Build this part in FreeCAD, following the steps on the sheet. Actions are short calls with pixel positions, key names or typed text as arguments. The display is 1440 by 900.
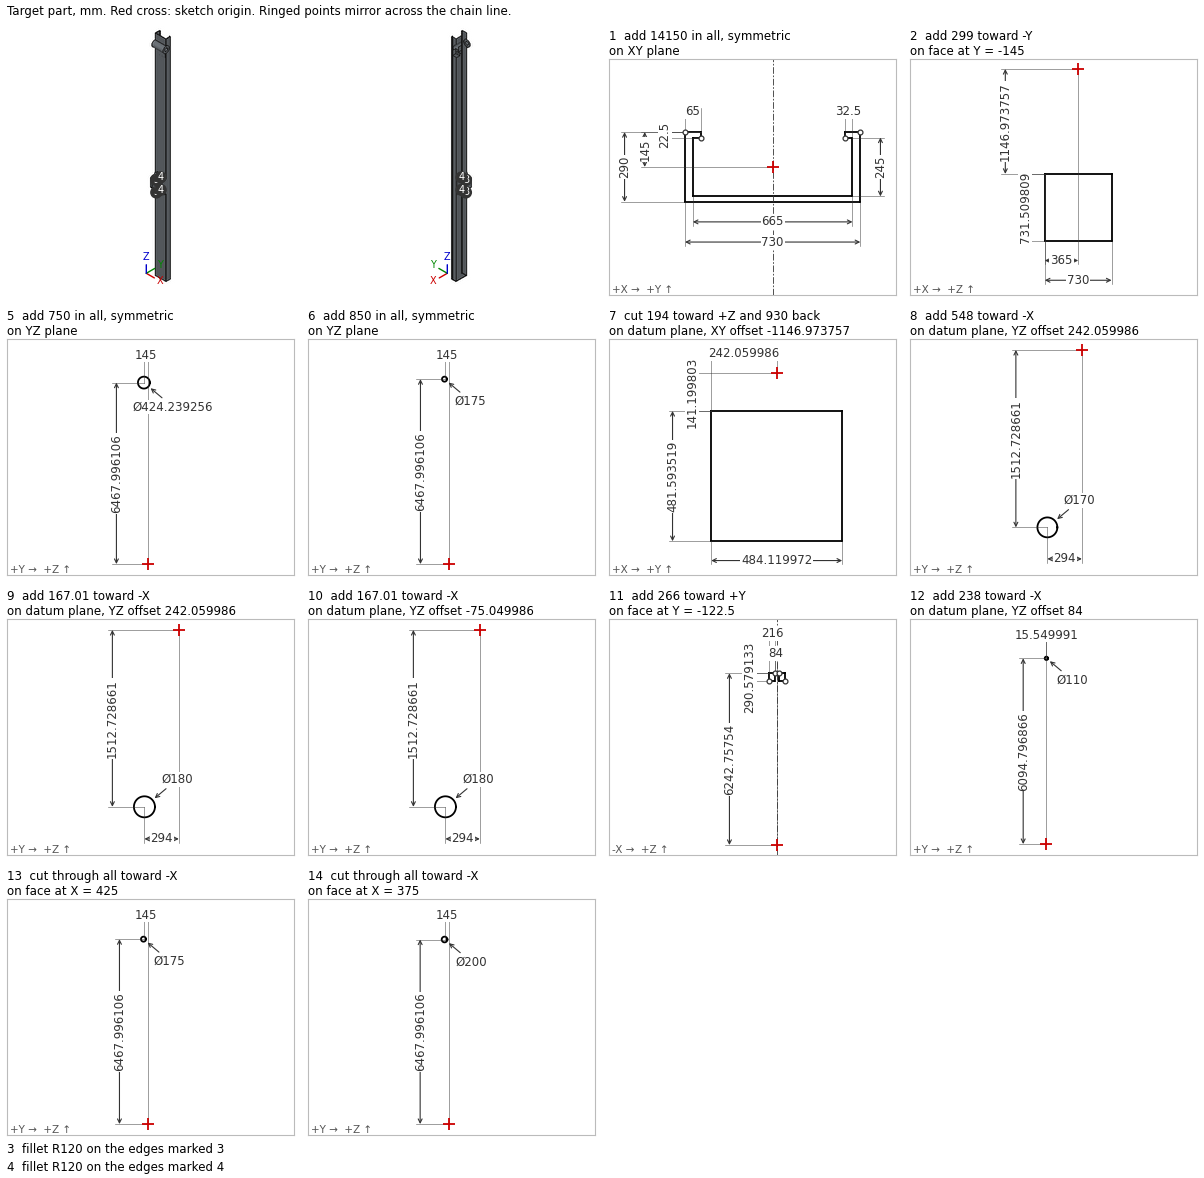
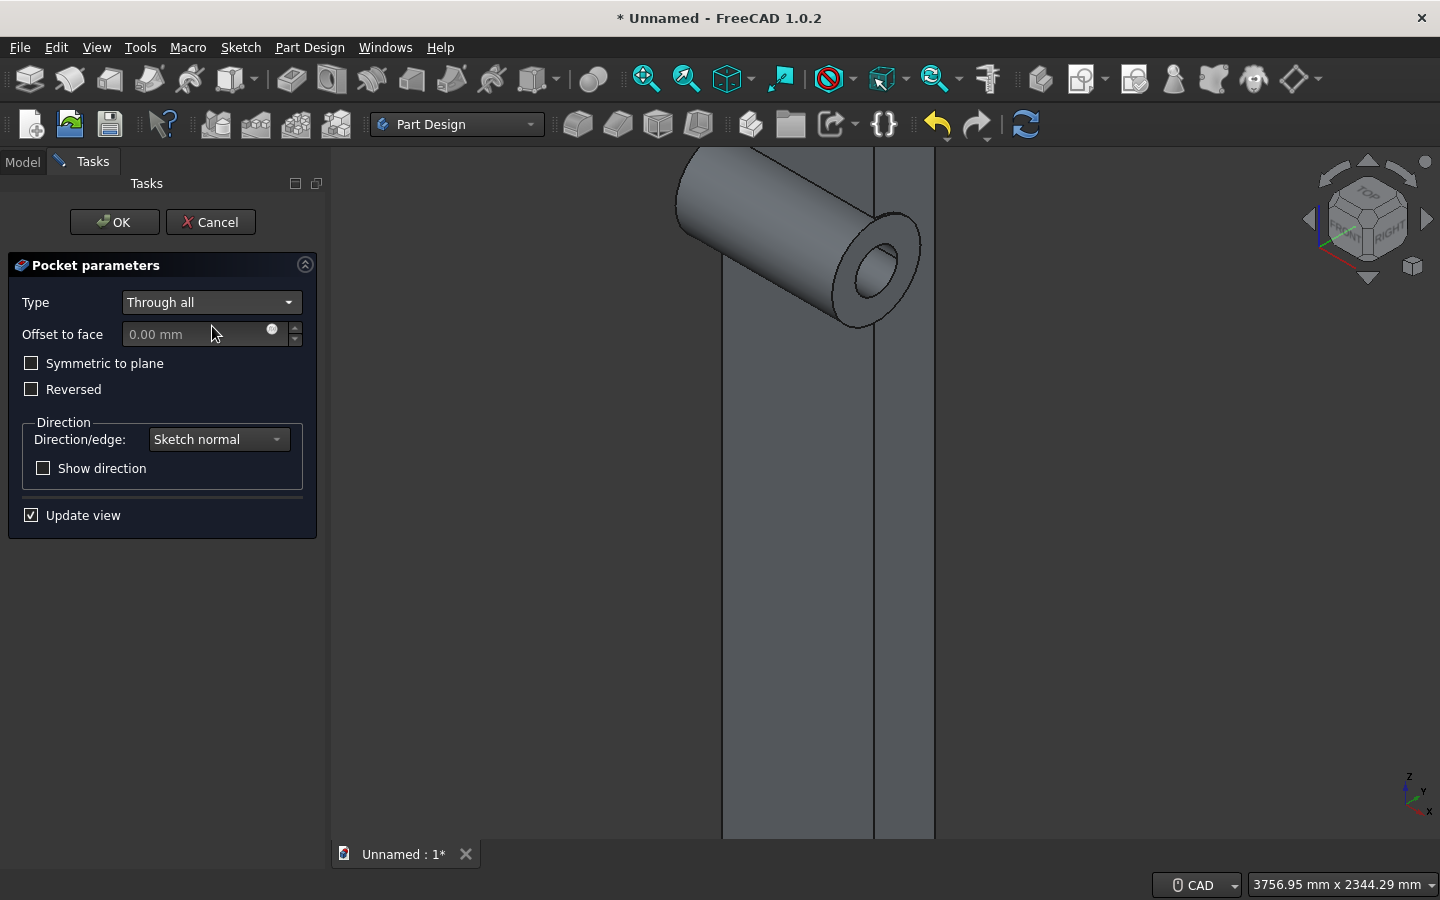
click(115, 222)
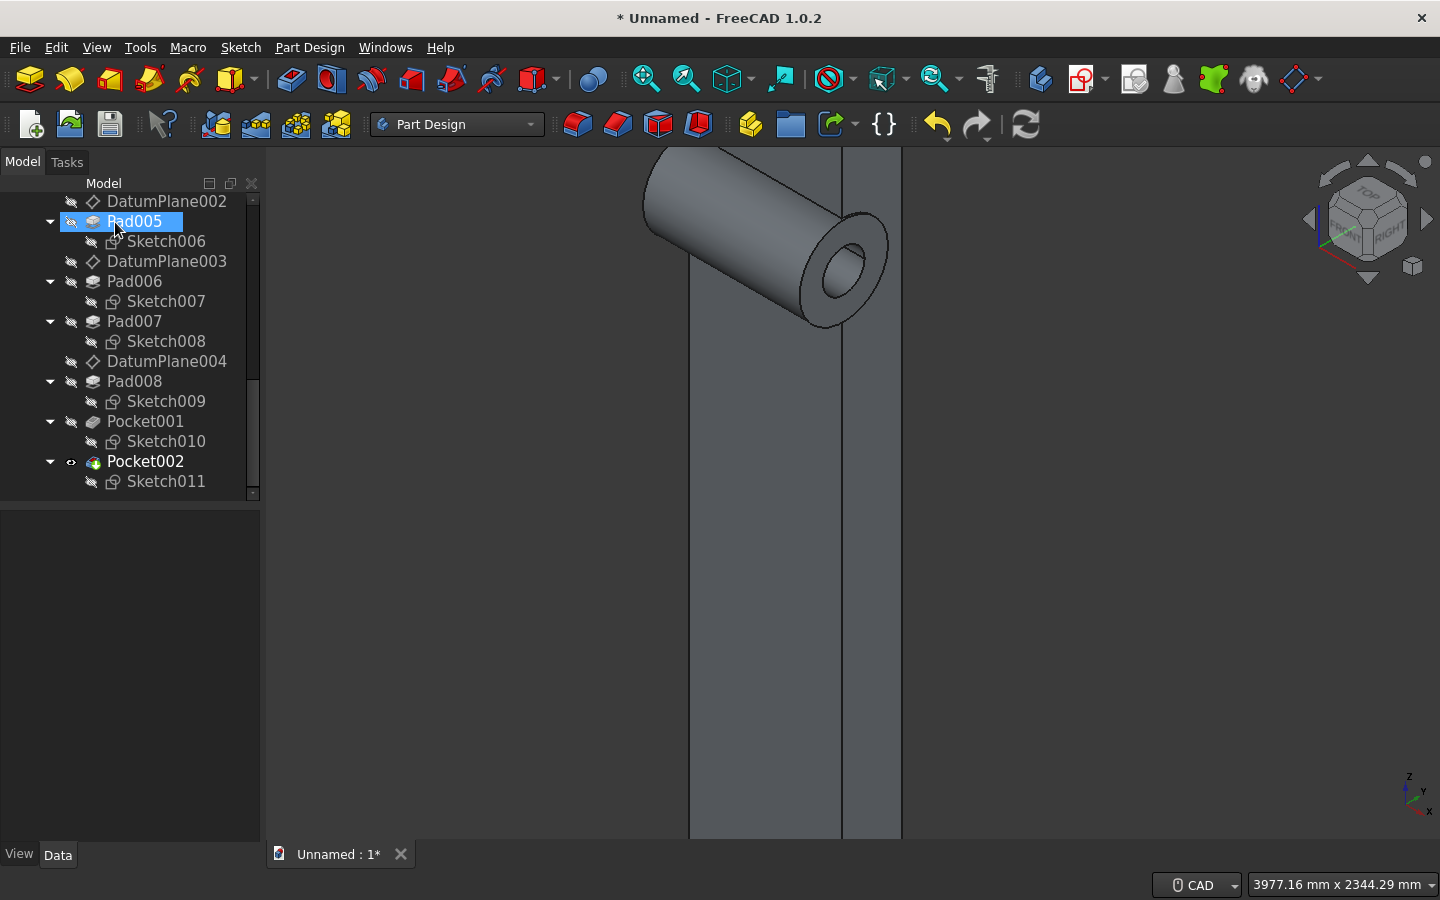
click(648, 80)